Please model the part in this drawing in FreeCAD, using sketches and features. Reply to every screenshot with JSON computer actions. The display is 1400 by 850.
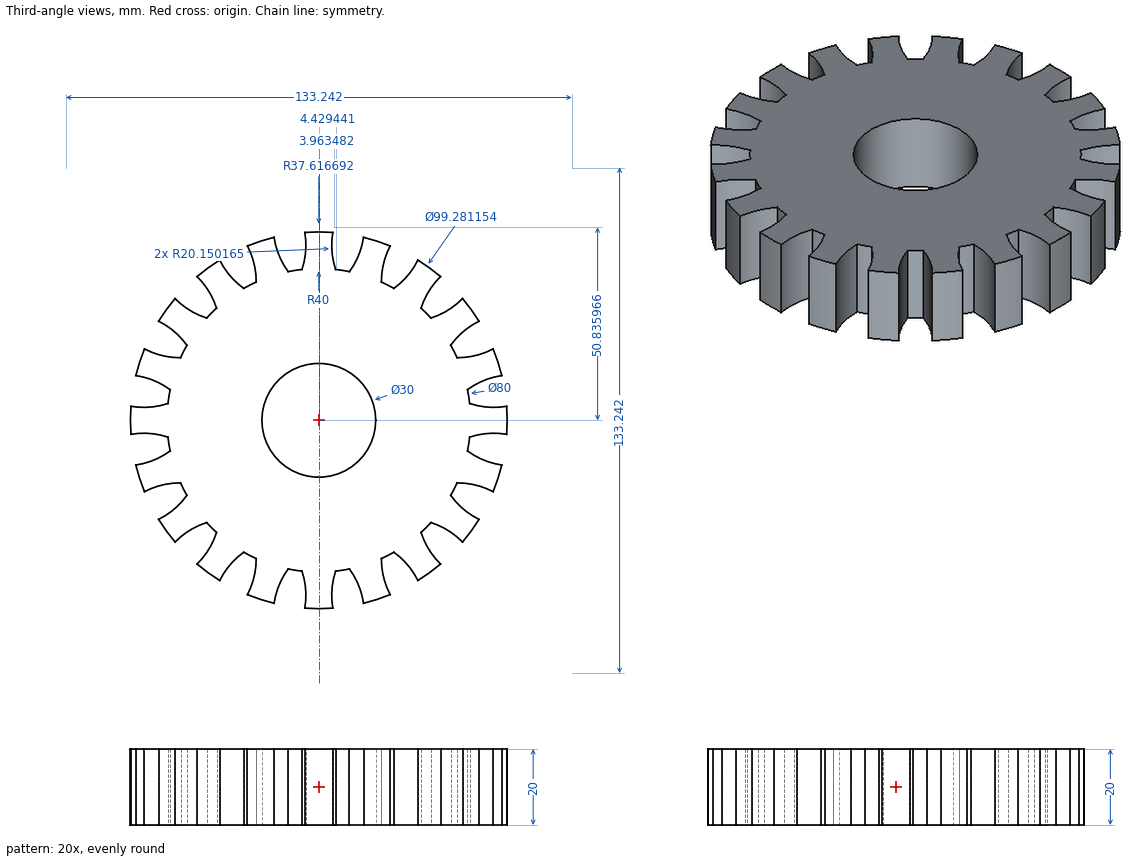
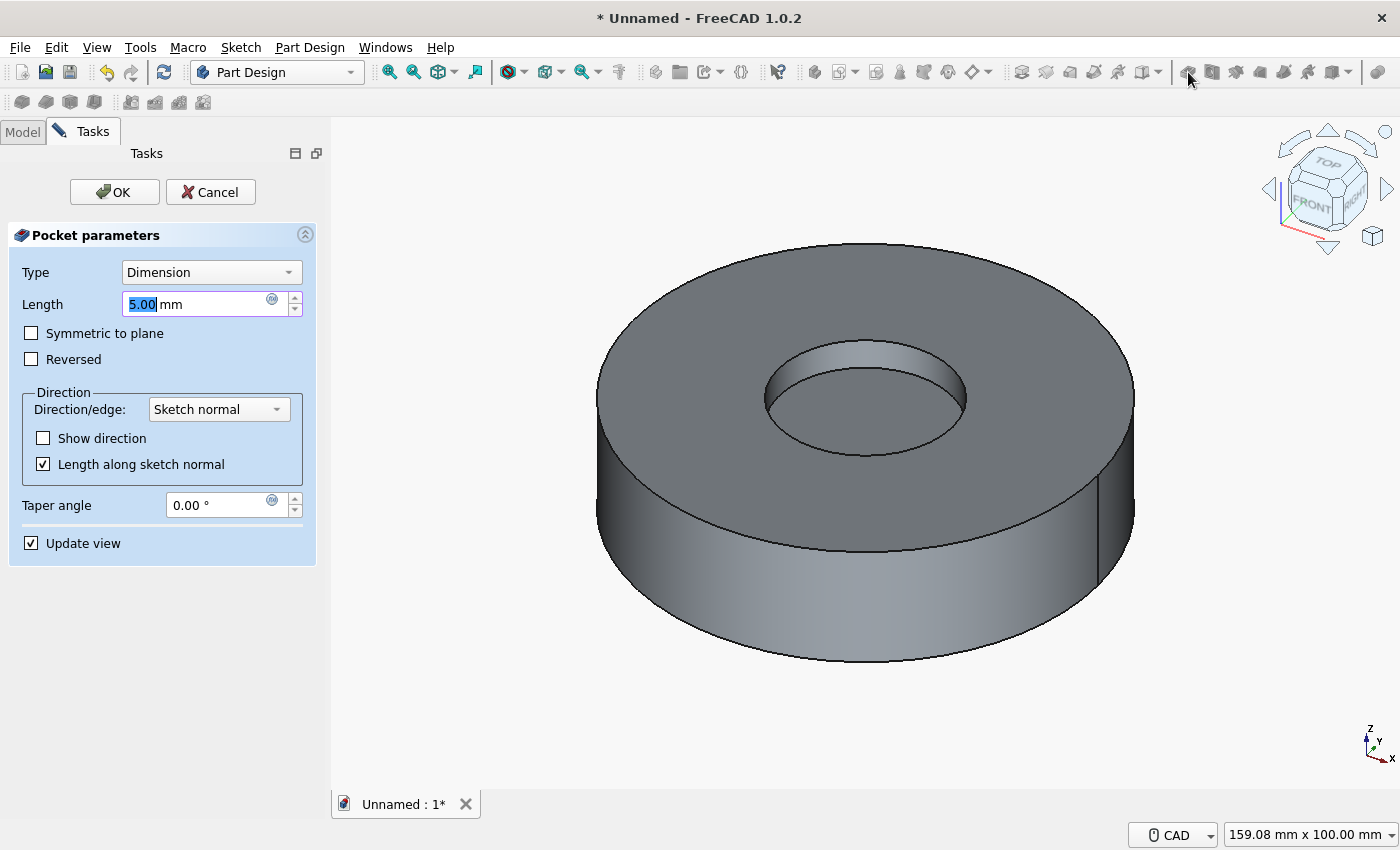
{"action": "left_click", "coordinate": [212, 272]}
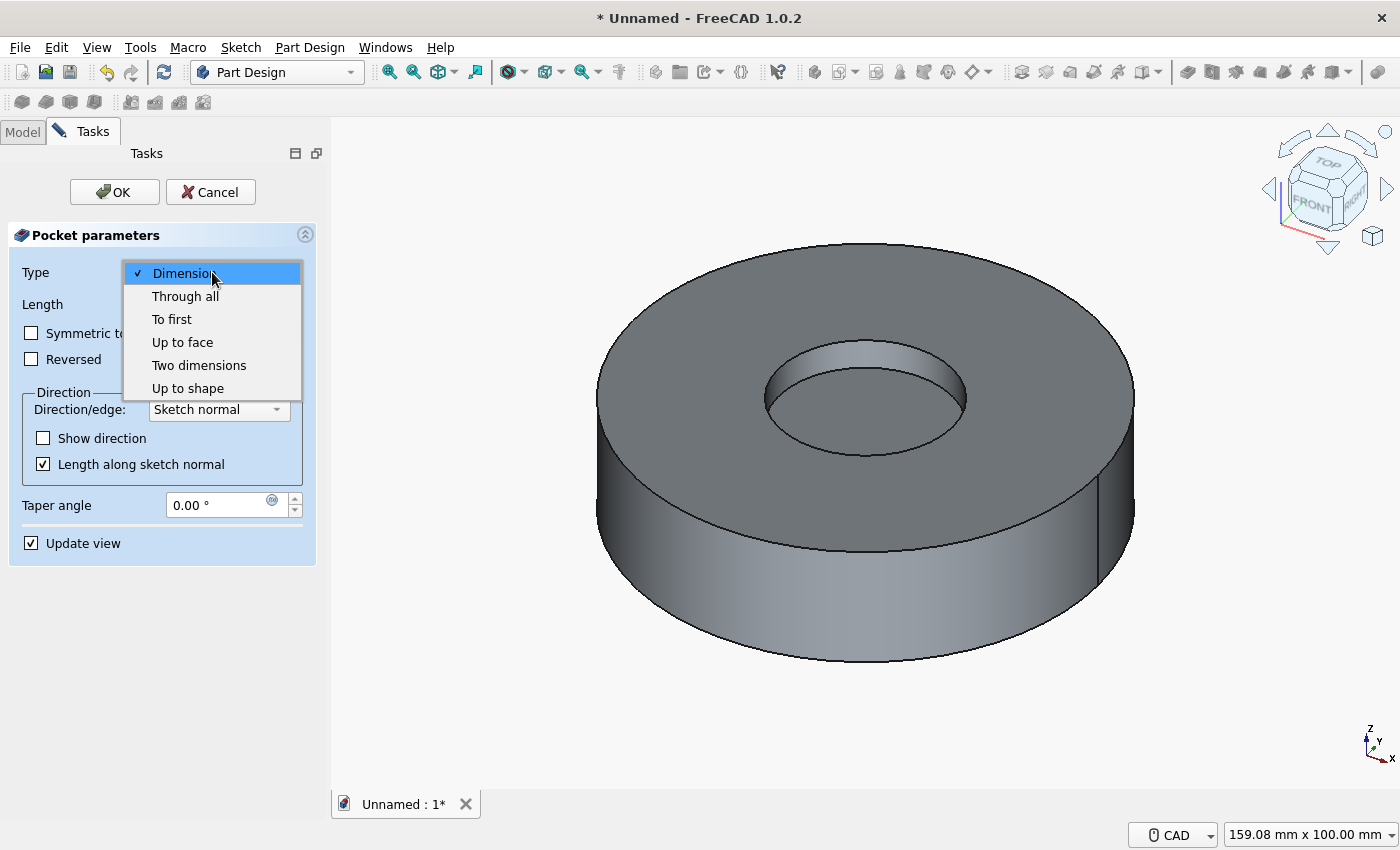
{"action": "left_click", "coordinate": [212, 320]}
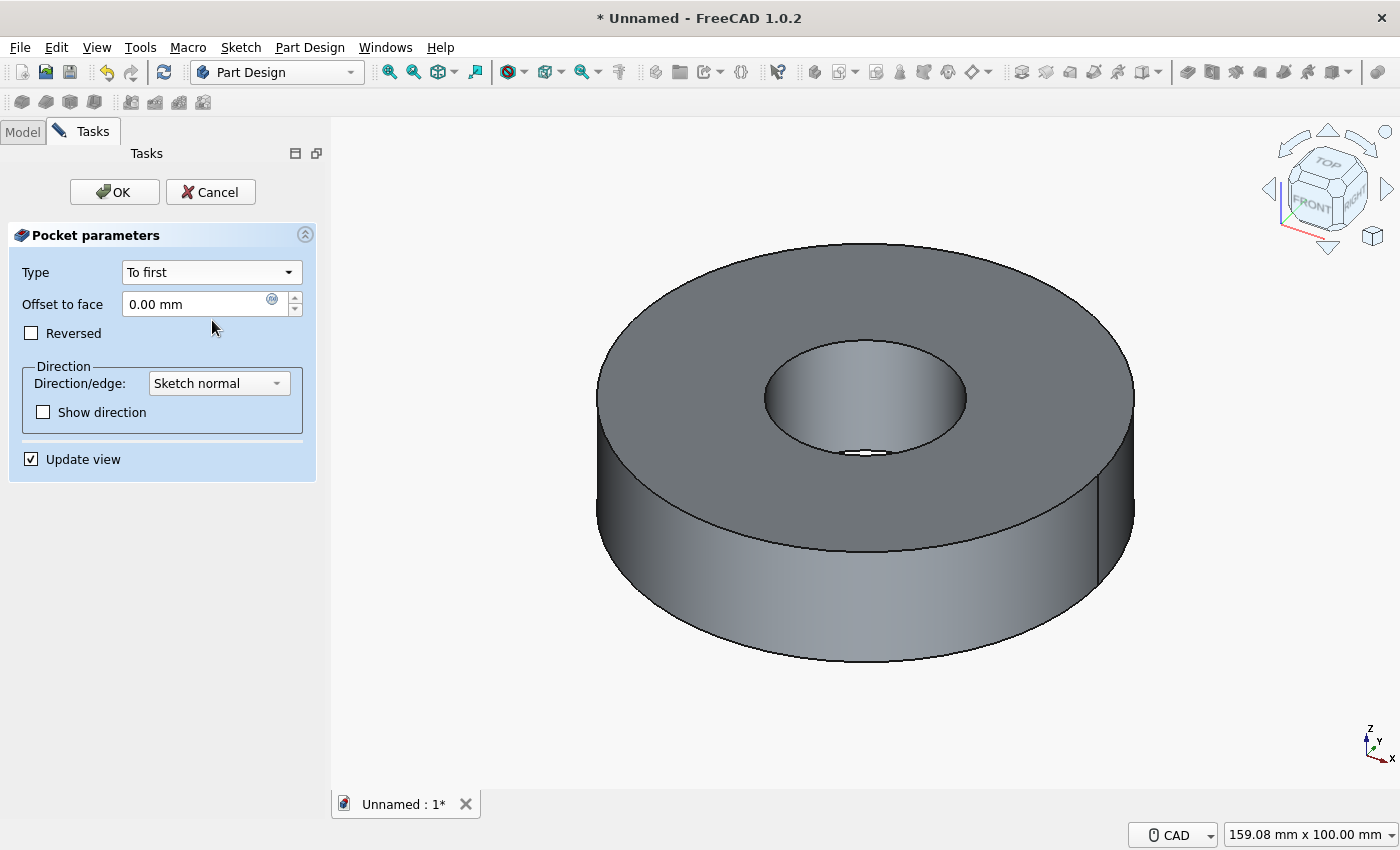
{"action": "left_click", "coordinate": [115, 192]}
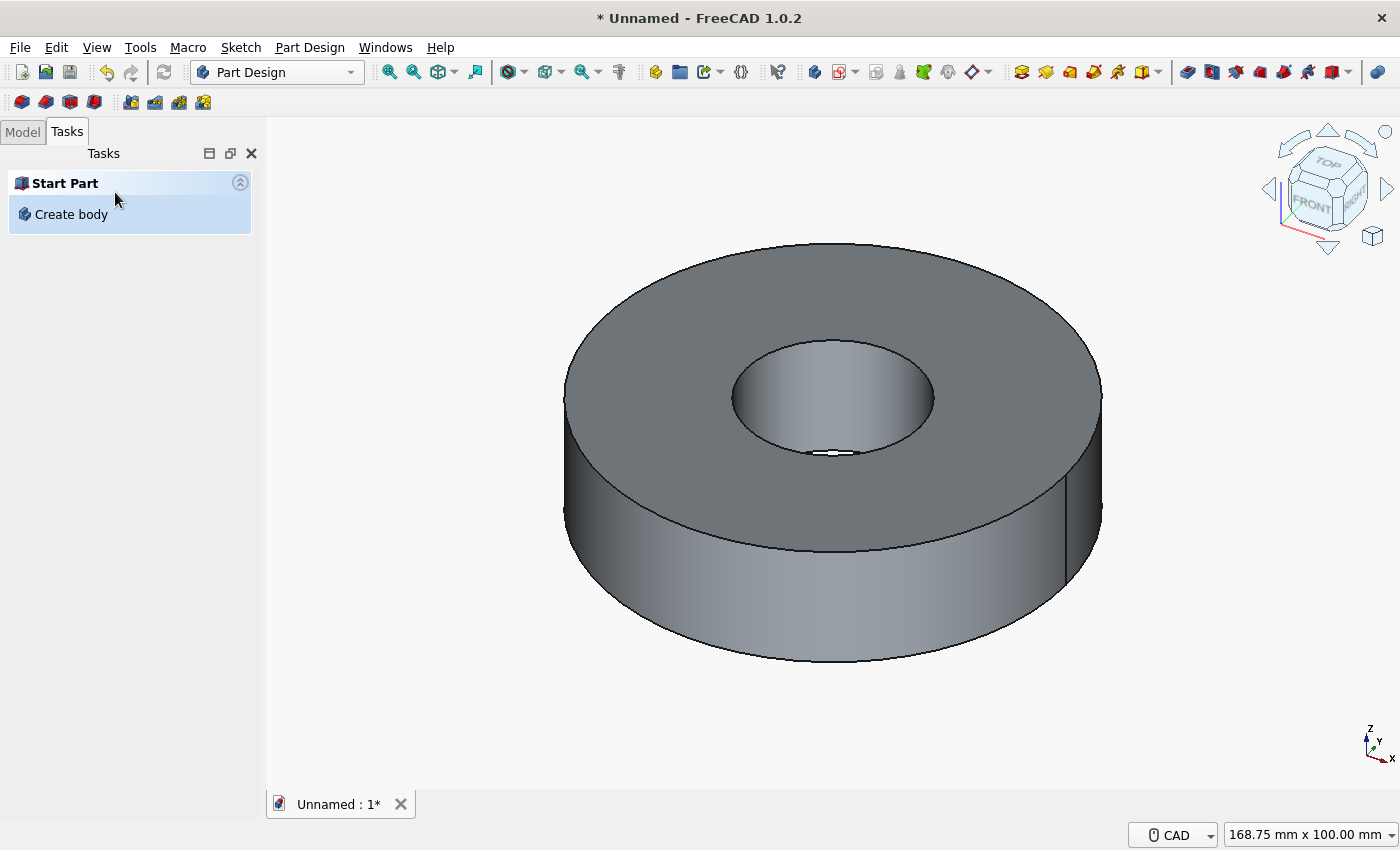
{"action": "left_click", "coordinate": [840, 72]}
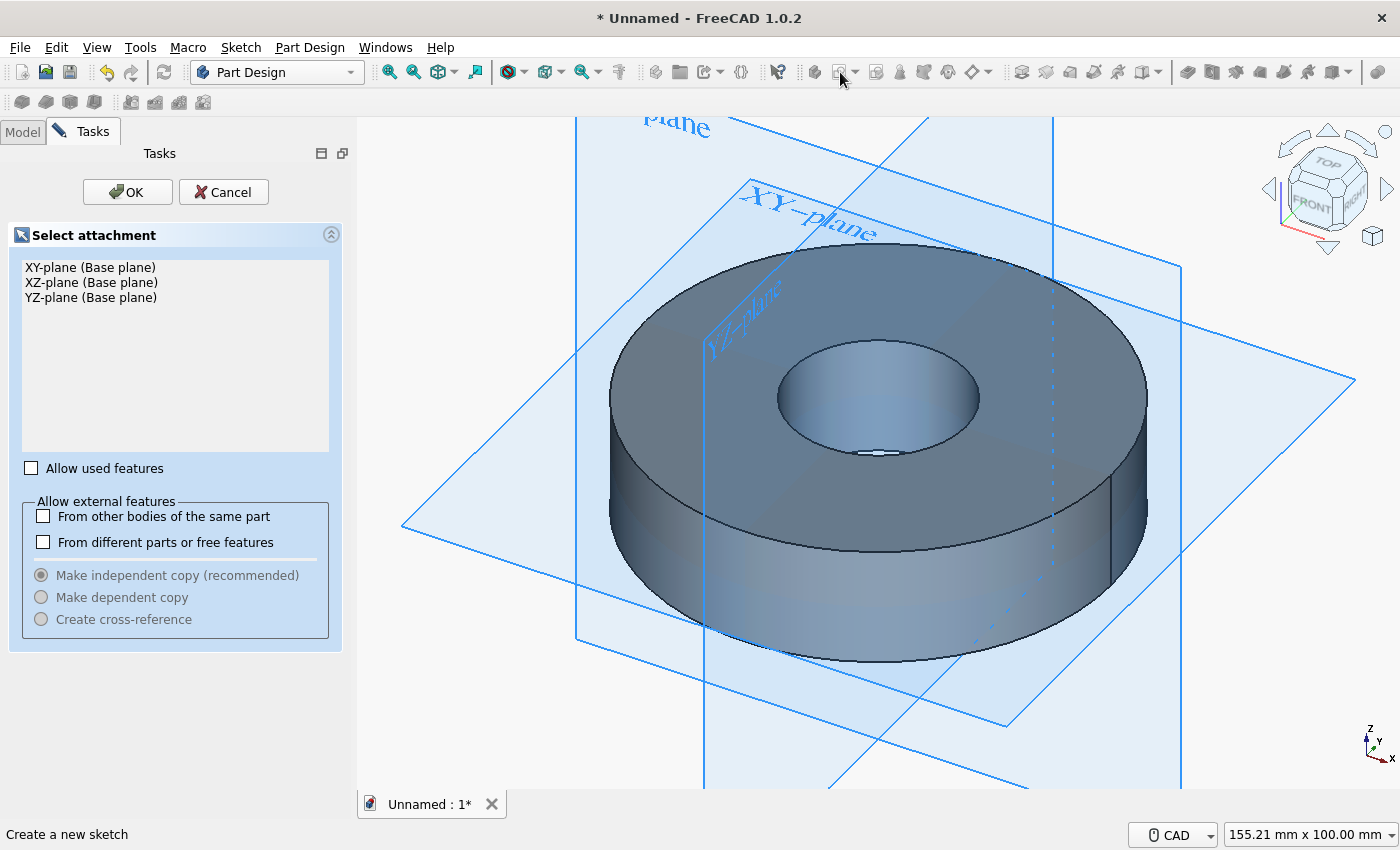
{"action": "left_click", "coordinate": [82, 268]}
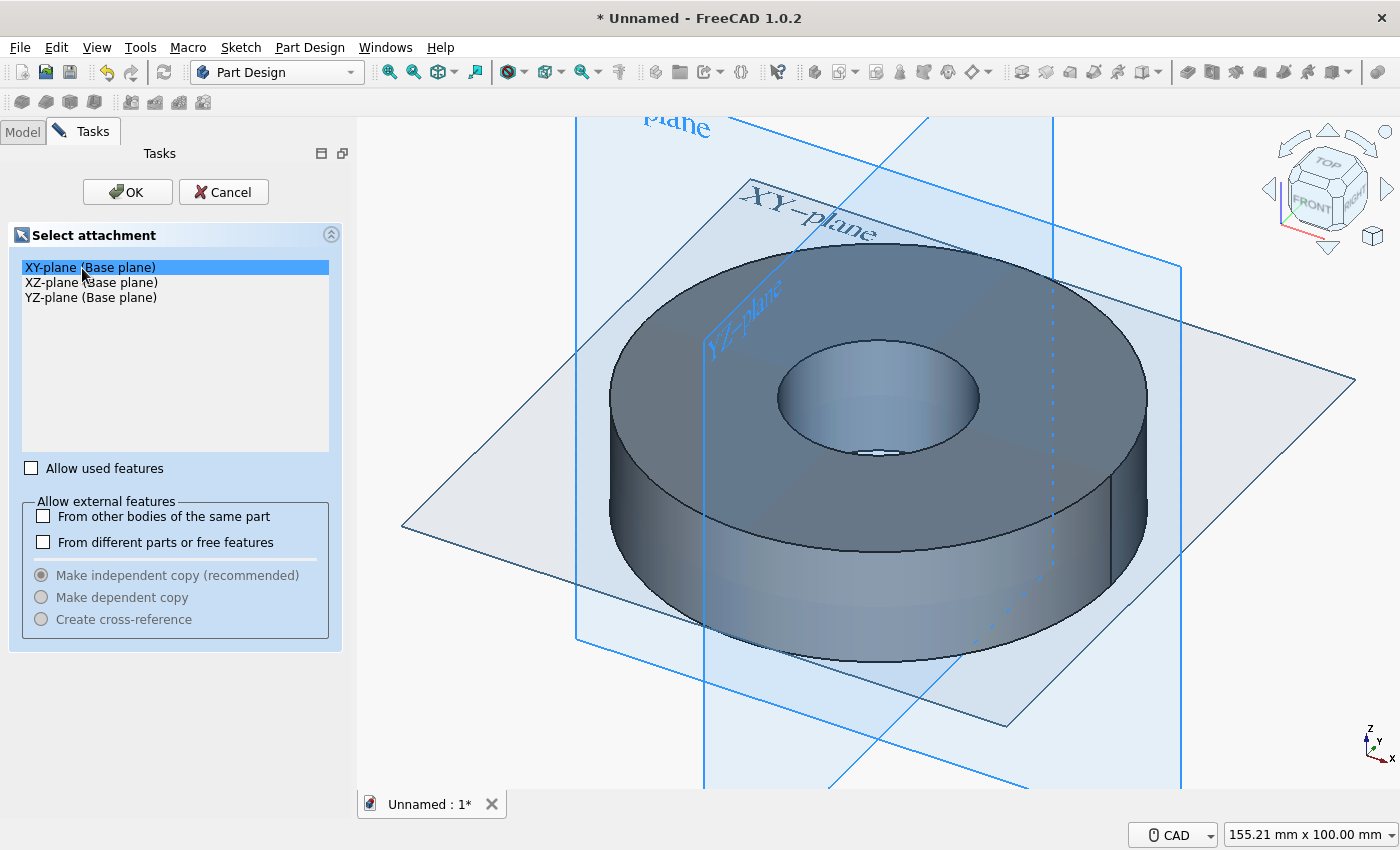
{"action": "left_click", "coordinate": [128, 192]}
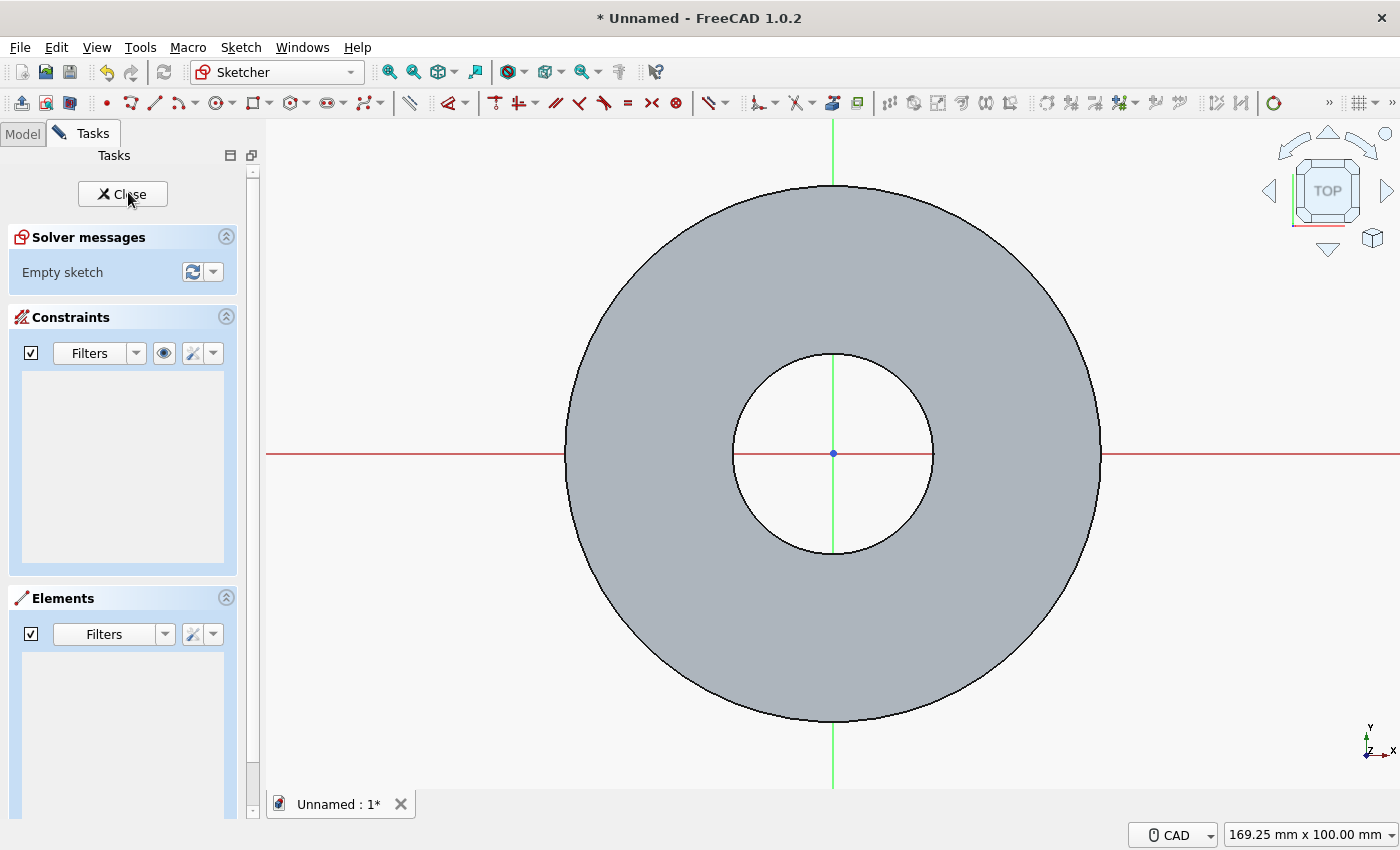
{"action": "left_click", "coordinate": [70, 104]}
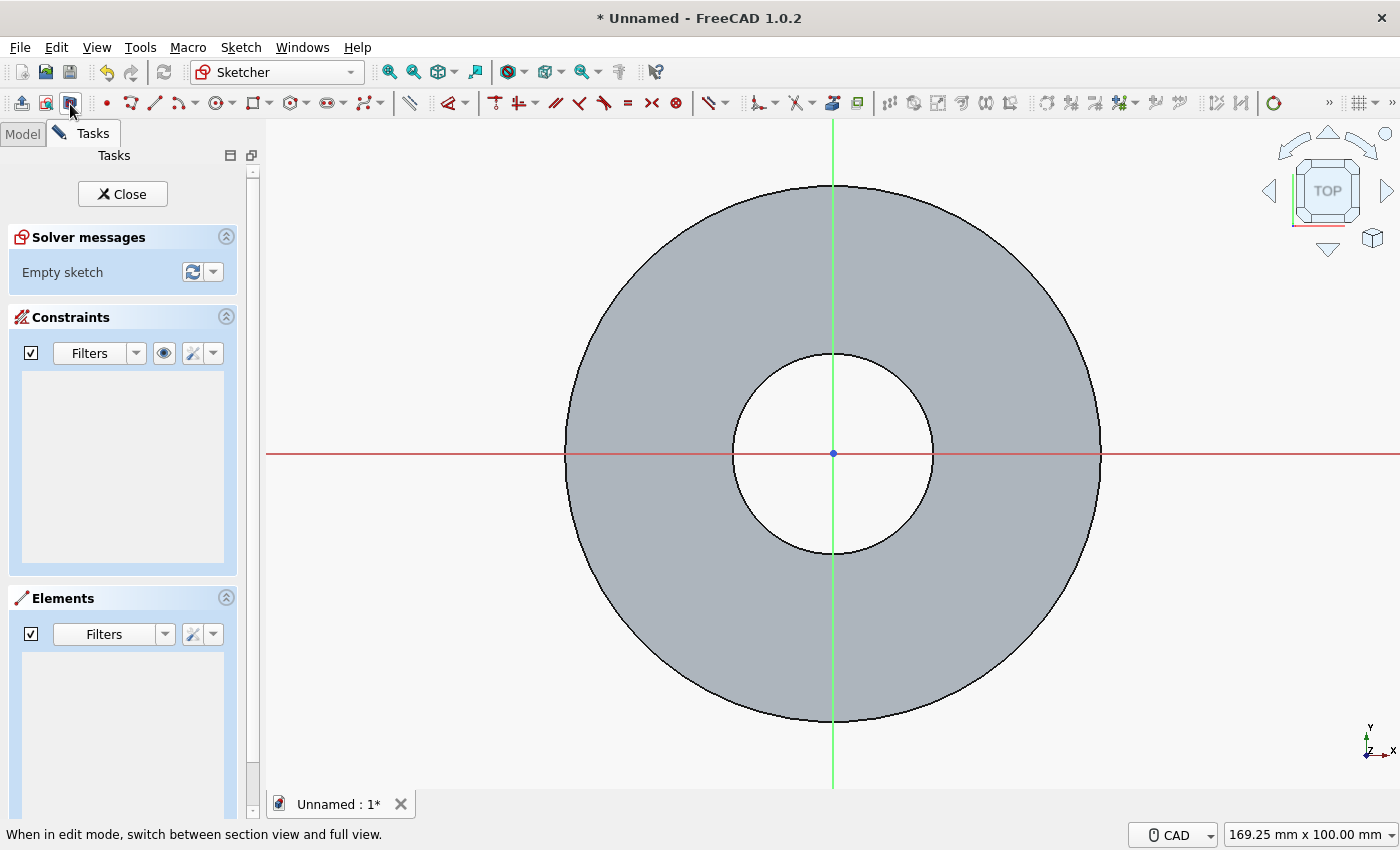
{"action": "scroll", "coordinate": [764, 454], "scroll_direction": "down", "scroll_amount": 5}